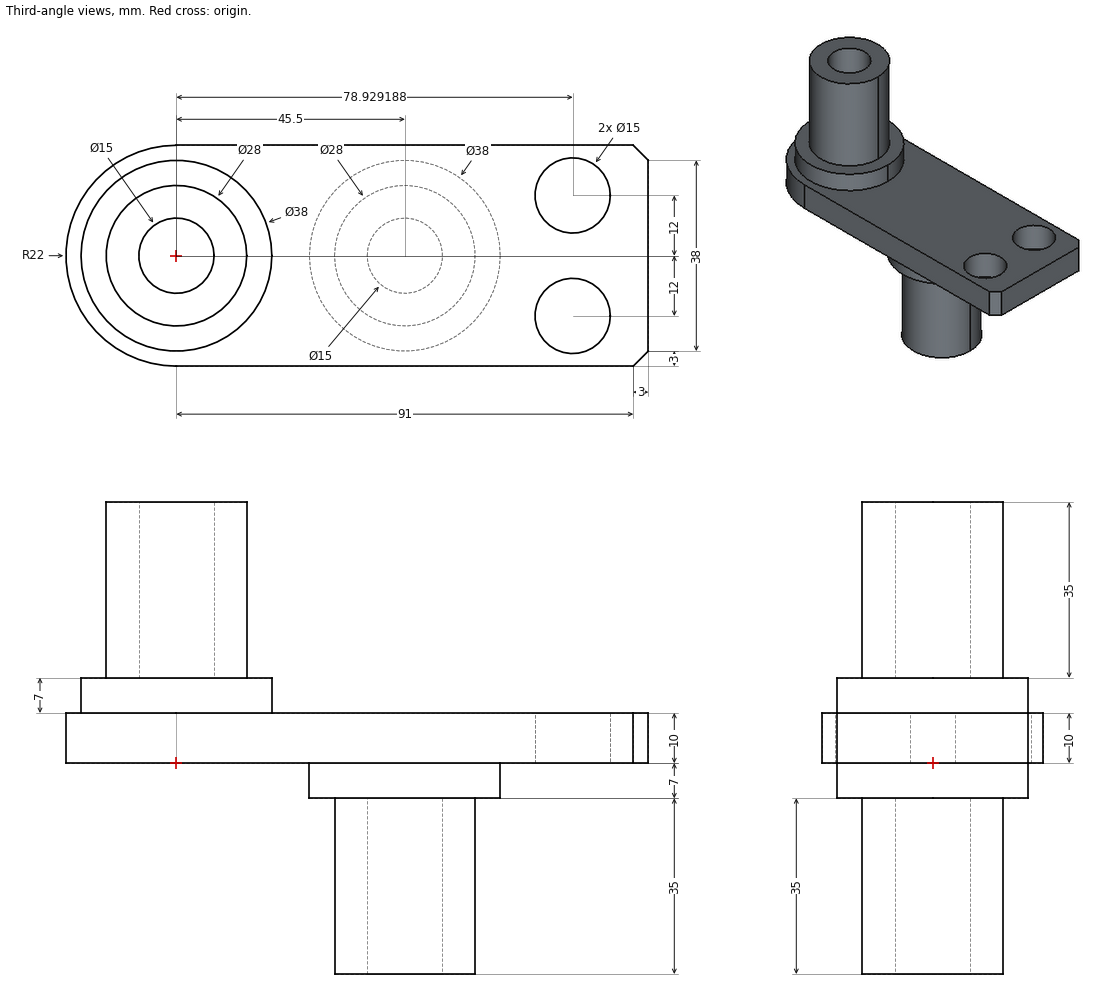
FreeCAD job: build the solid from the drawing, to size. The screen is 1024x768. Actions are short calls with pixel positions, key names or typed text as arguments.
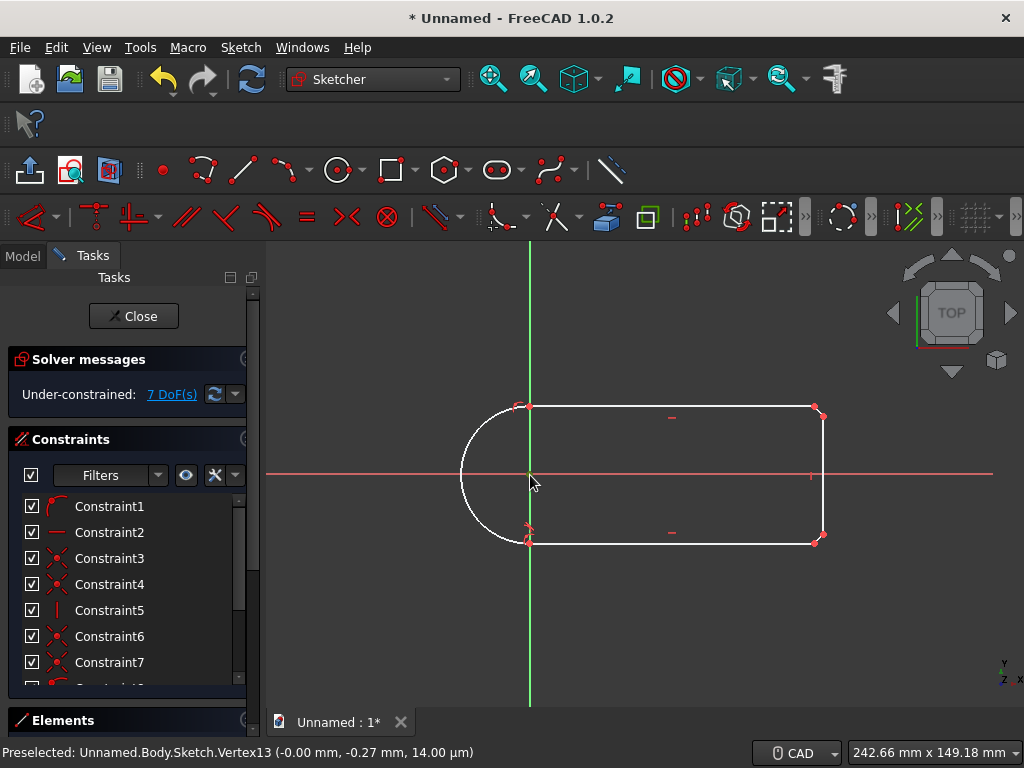
click(334, 474)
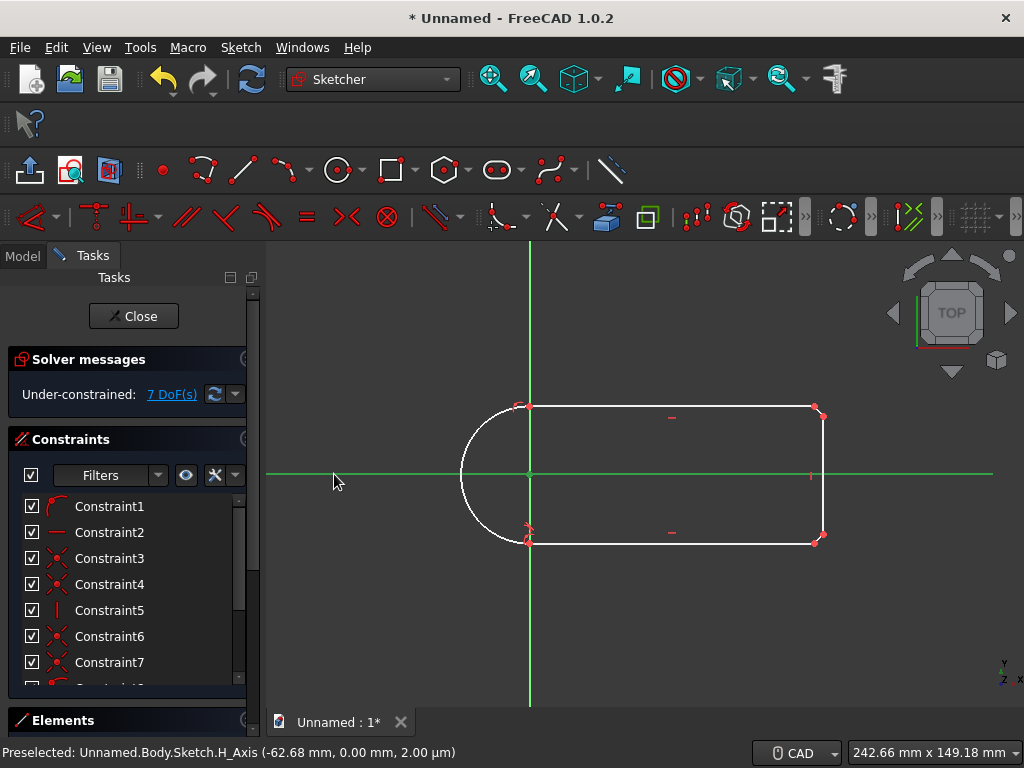
click(94, 218)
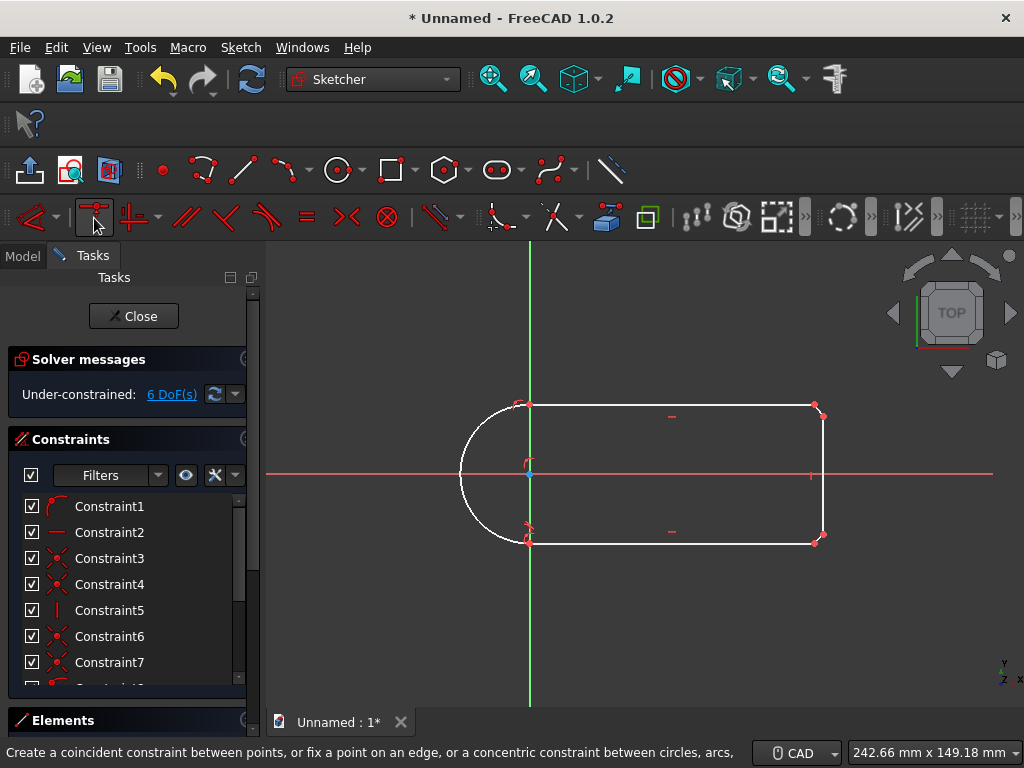
click(32, 218)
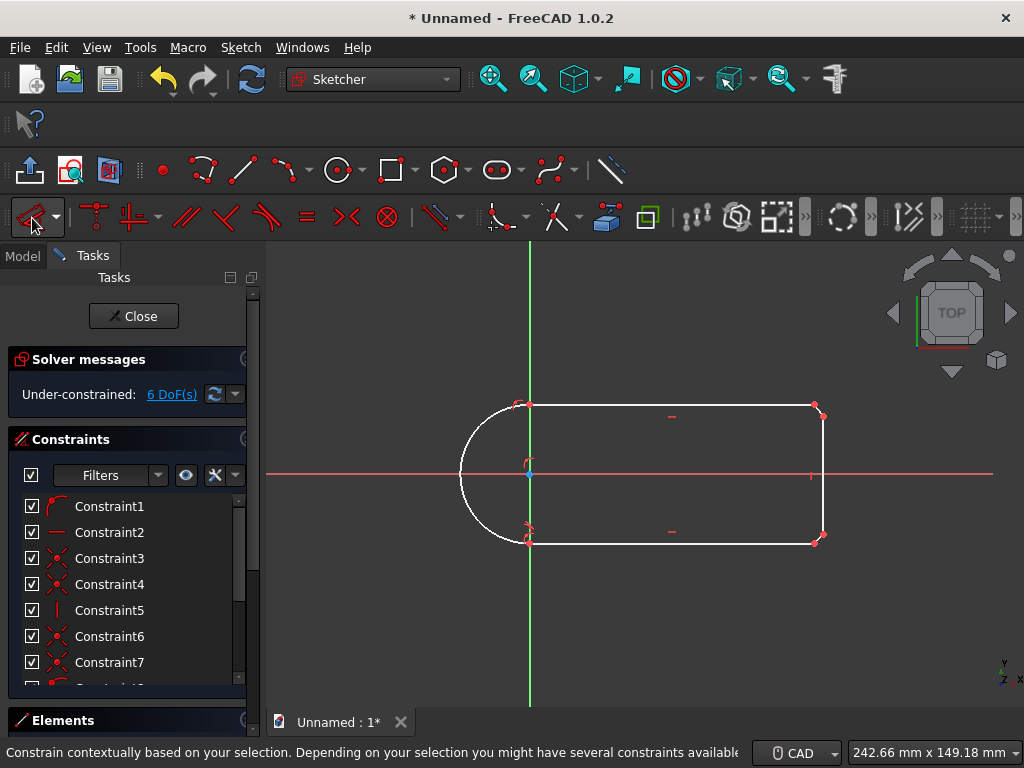
click(474, 433)
click(448, 414)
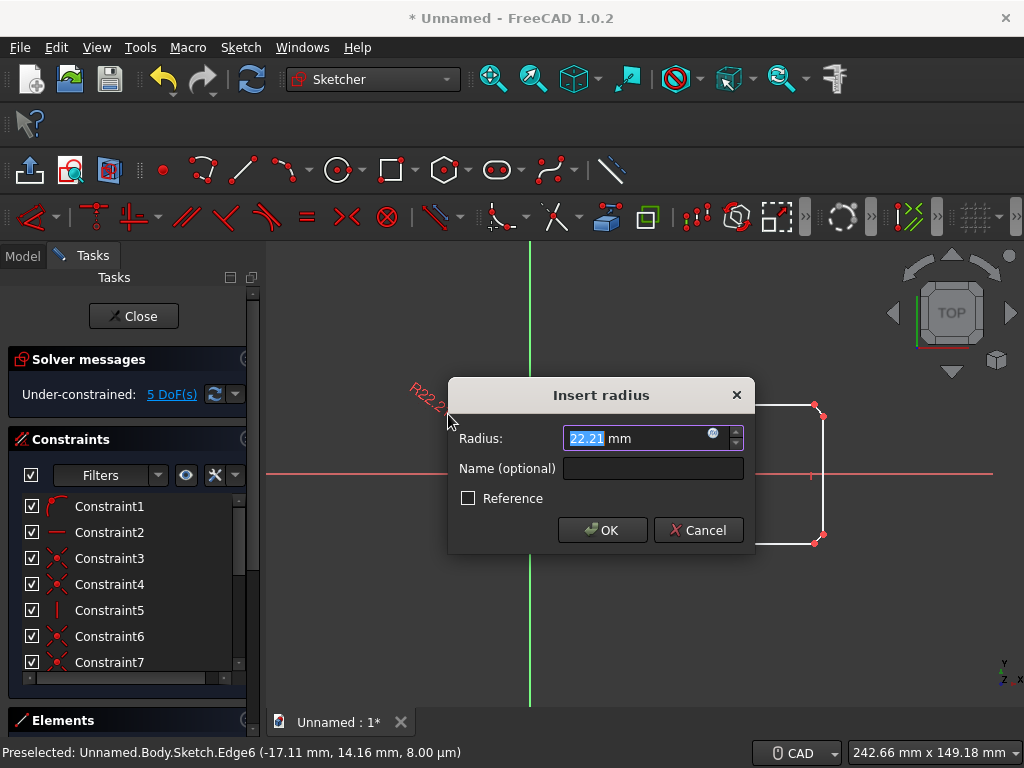
text(22)
key(Return)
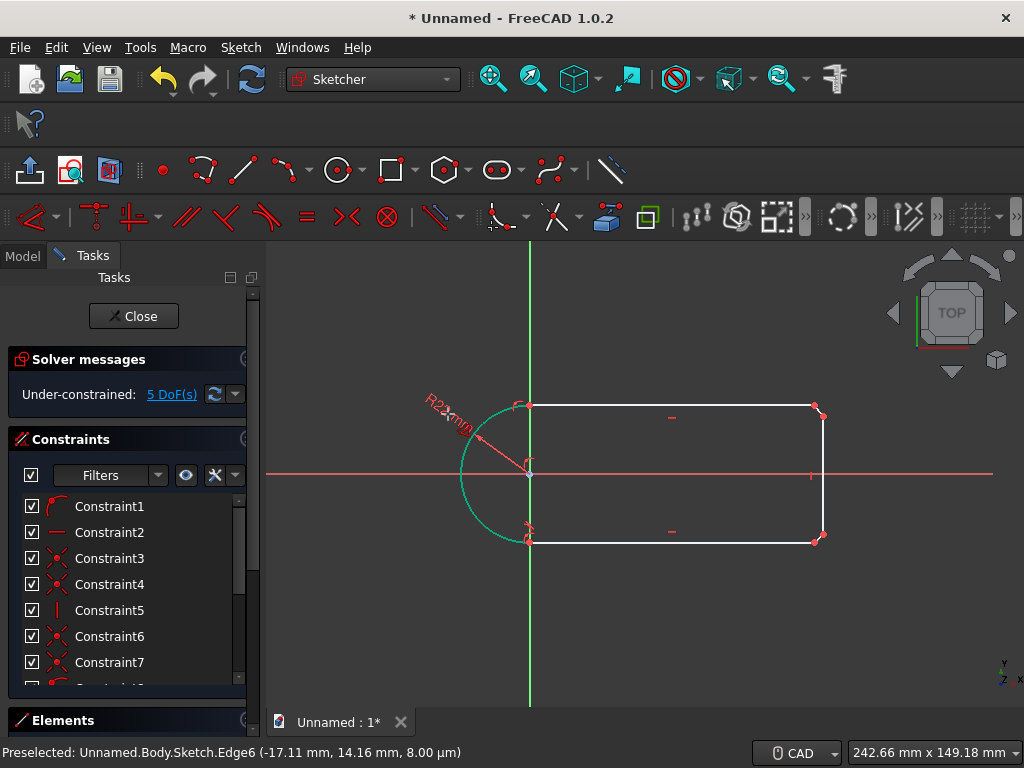
click(615, 543)
click(672, 577)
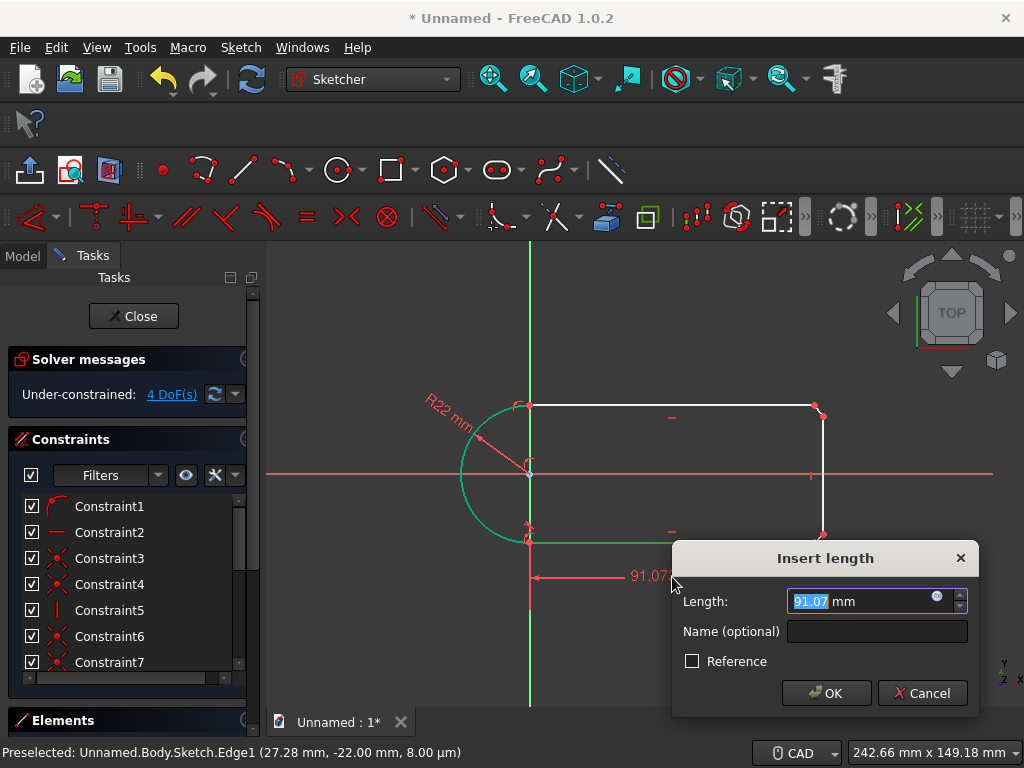
text(91)
key(Return)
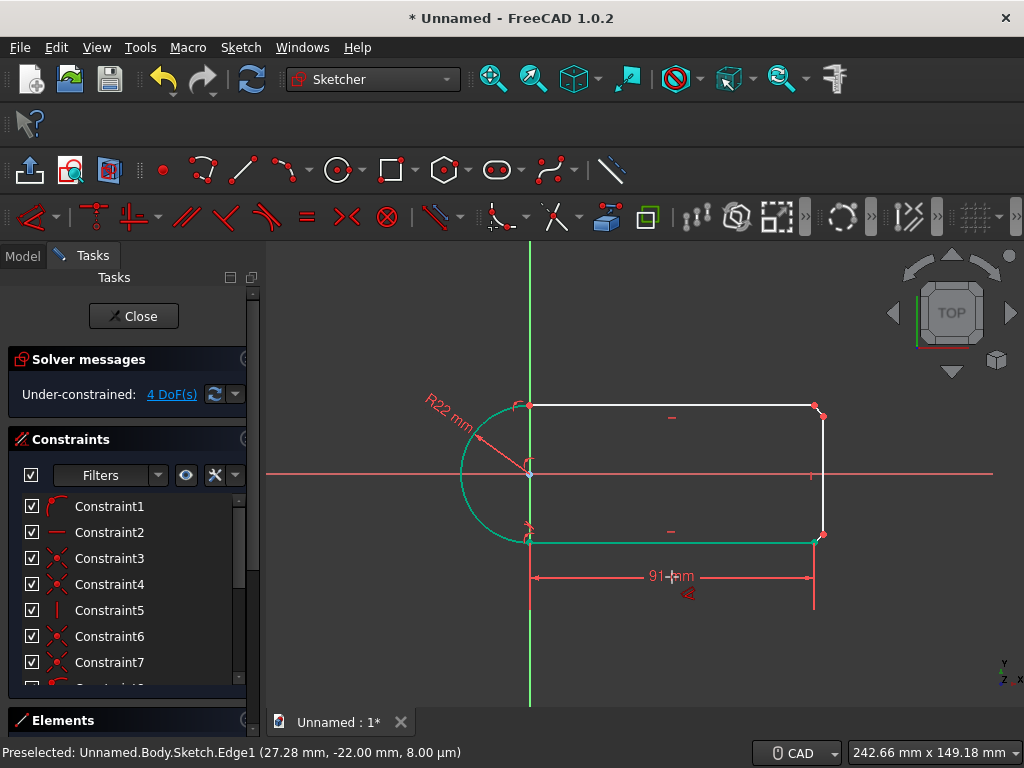
click(823, 499)
click(857, 448)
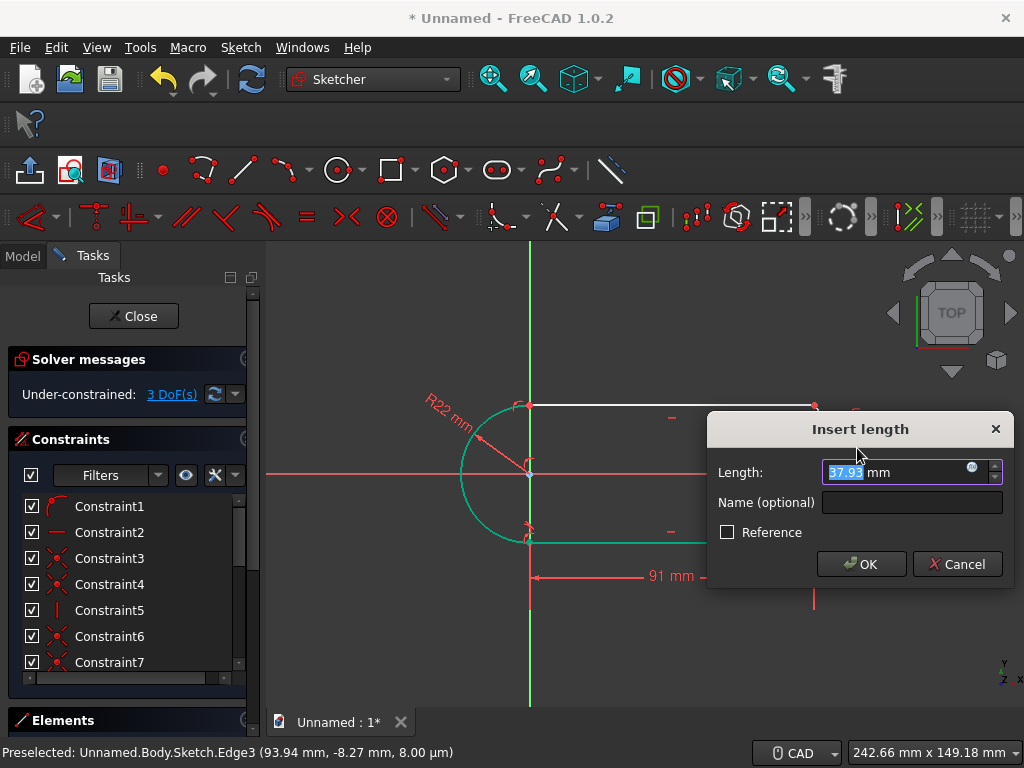
text(38)
key(Return)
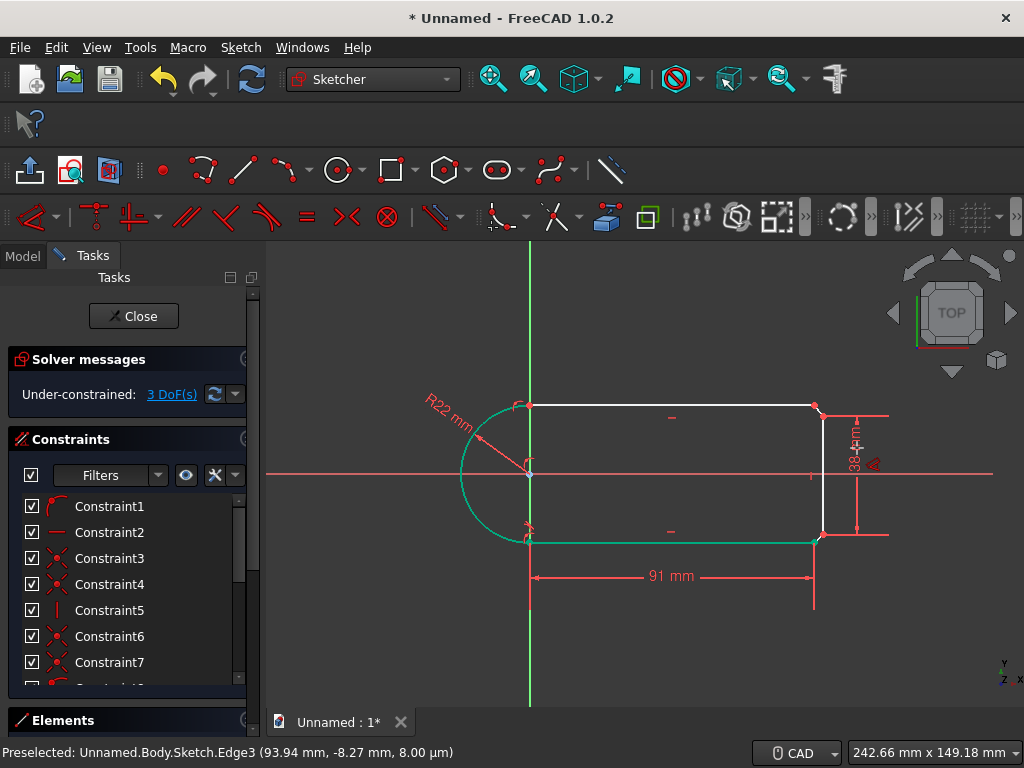
click(729, 405)
click(672, 371)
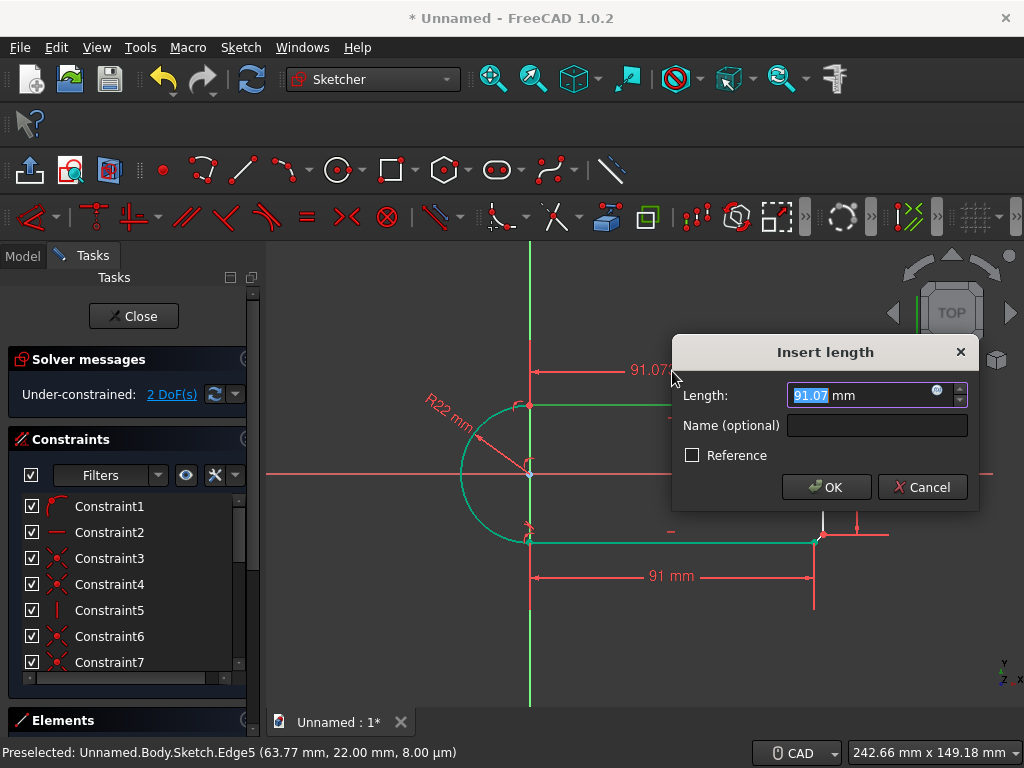
text(91)
key(Return)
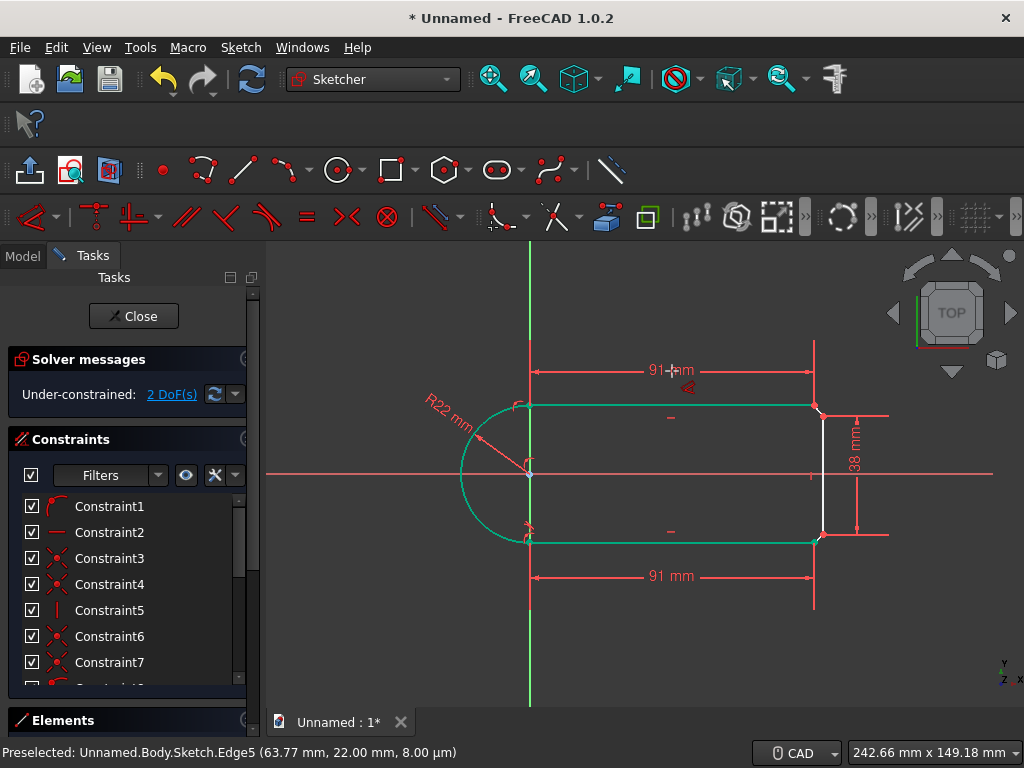
scroll(819, 539, up, 8)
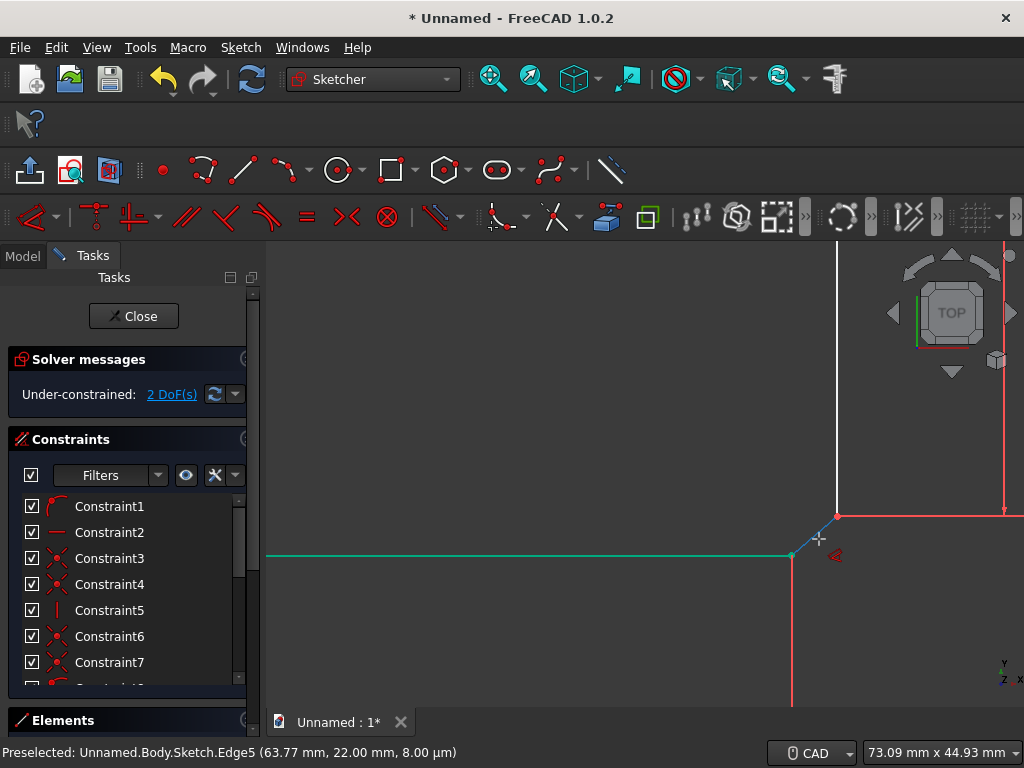
click(814, 536)
click(814, 590)